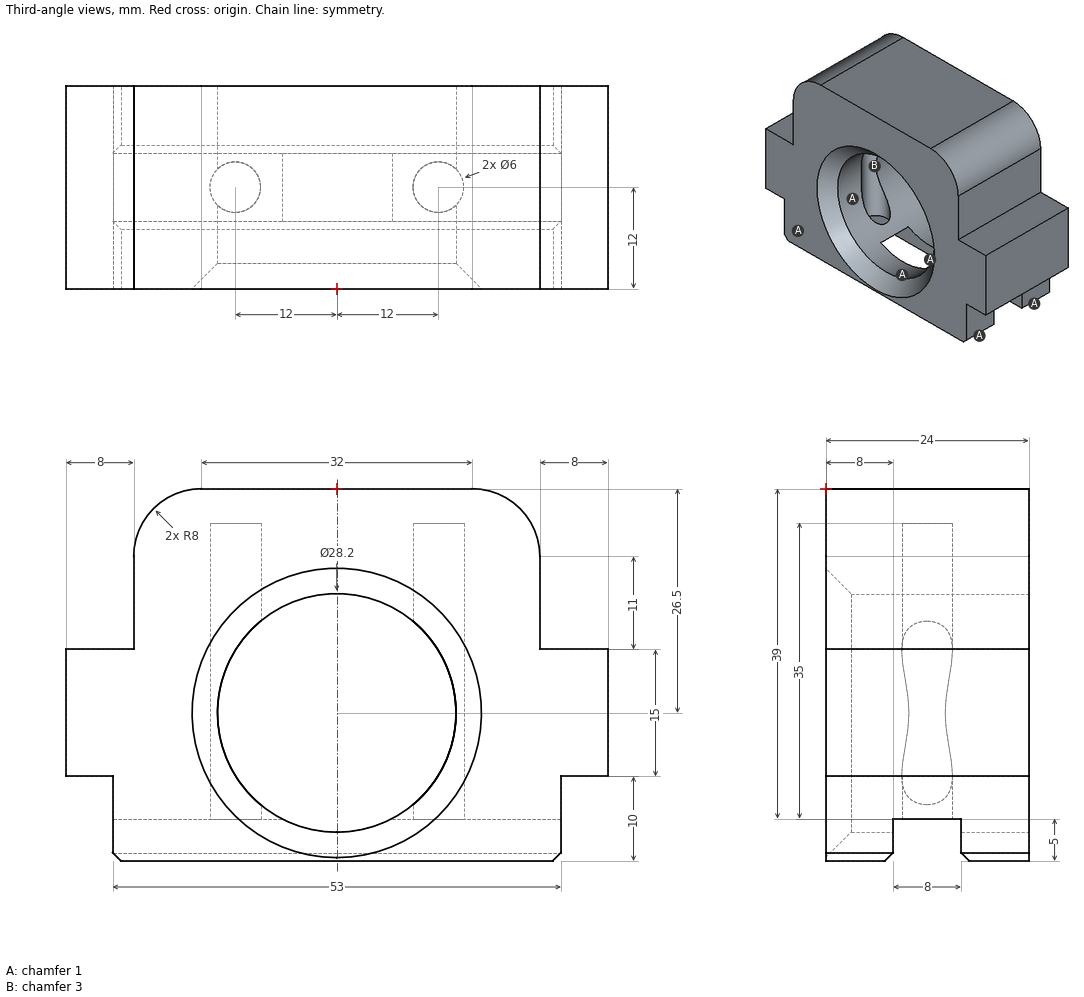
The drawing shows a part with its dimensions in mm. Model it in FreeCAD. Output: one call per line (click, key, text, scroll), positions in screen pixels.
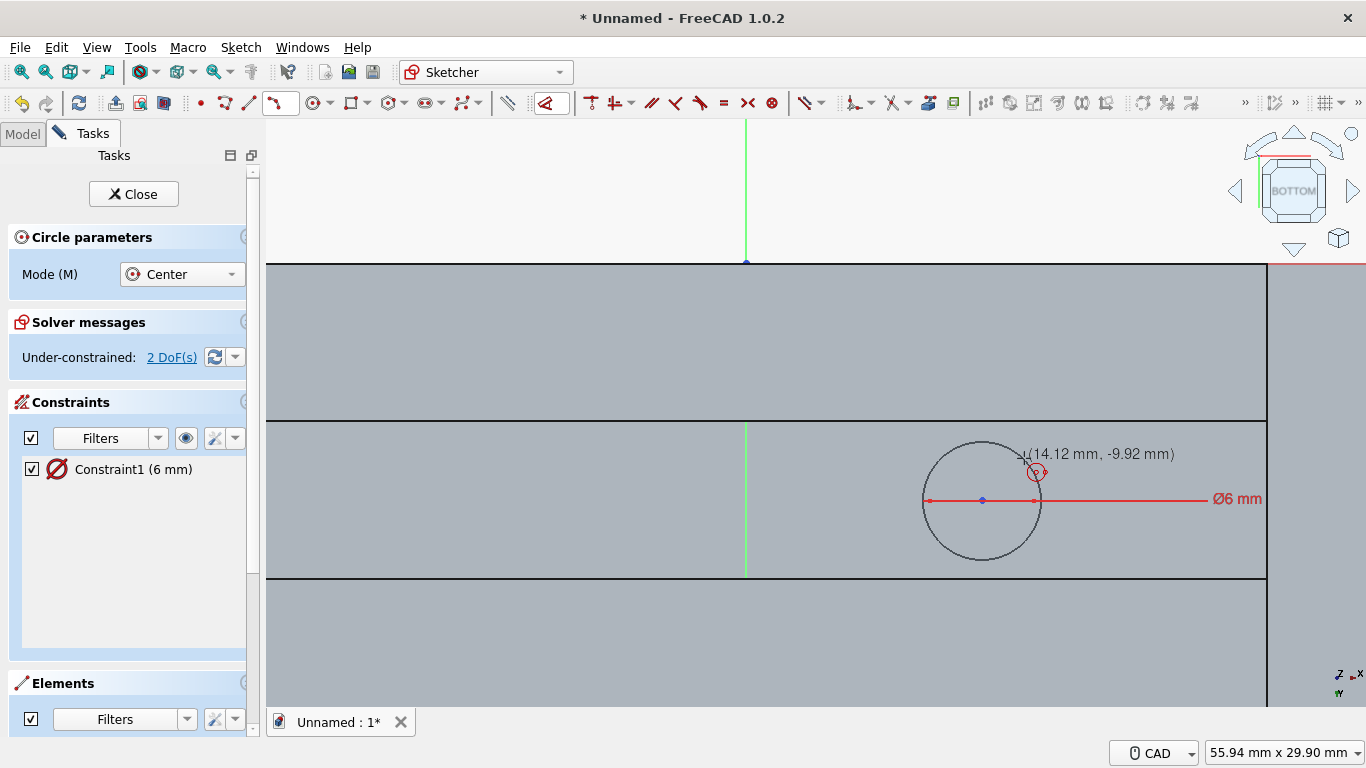
click(510, 500)
move(552, 458)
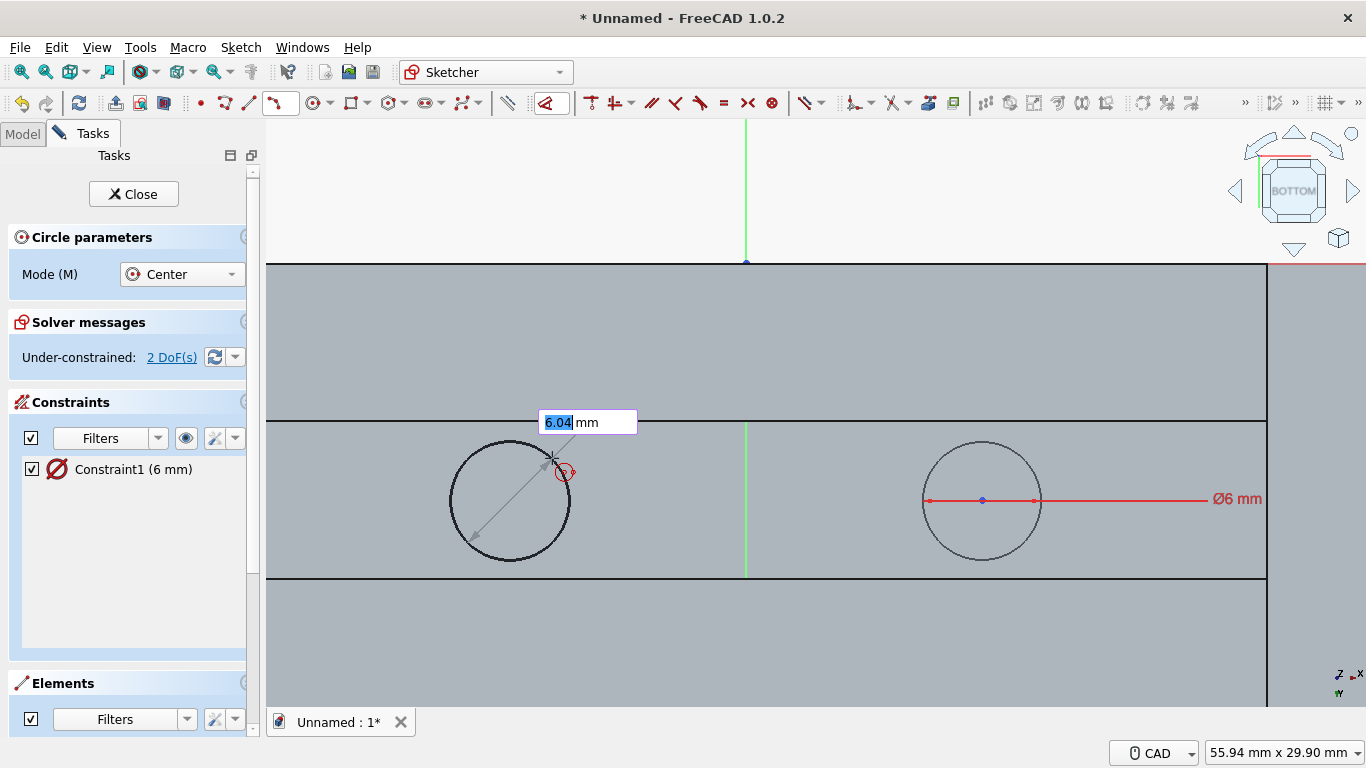
text(6)
key(Return)
key(Escape)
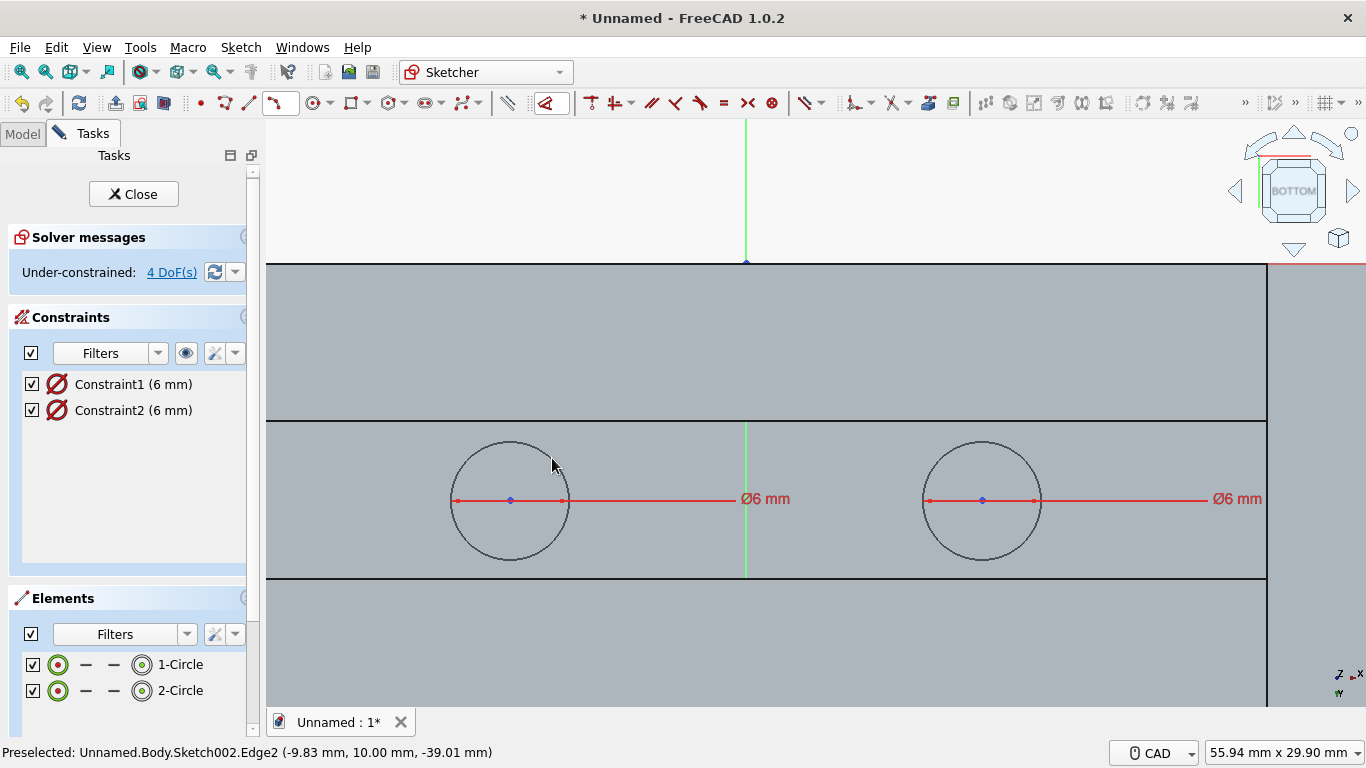
click(982, 501)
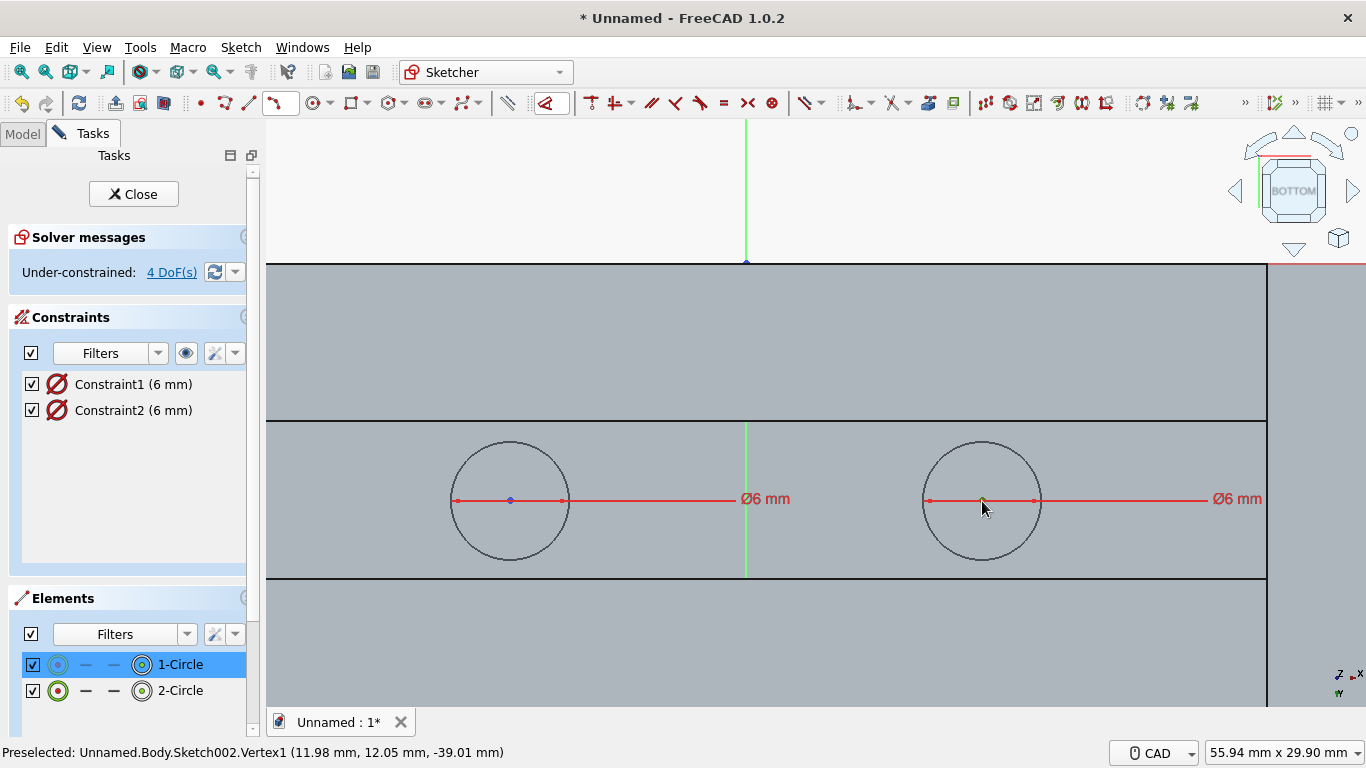
click(510, 501)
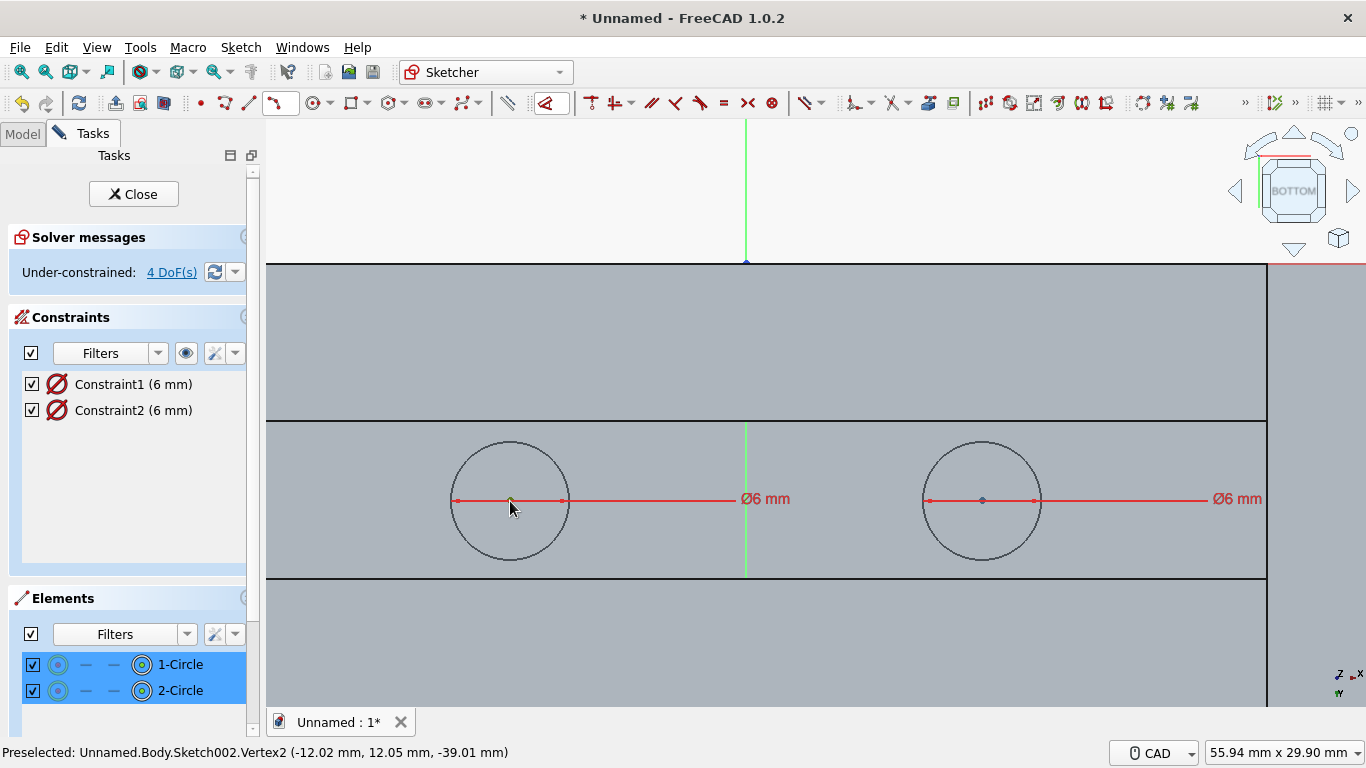
click(634, 104)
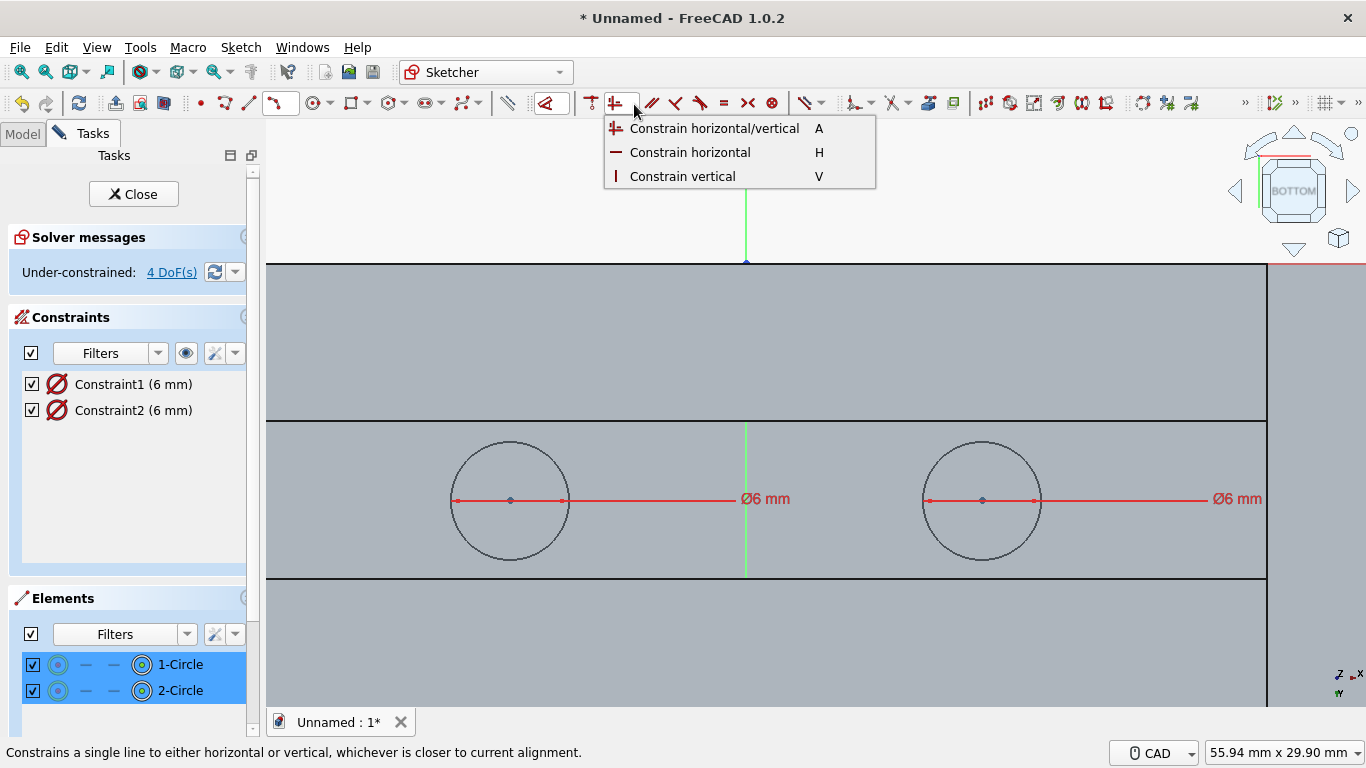
click(740, 152)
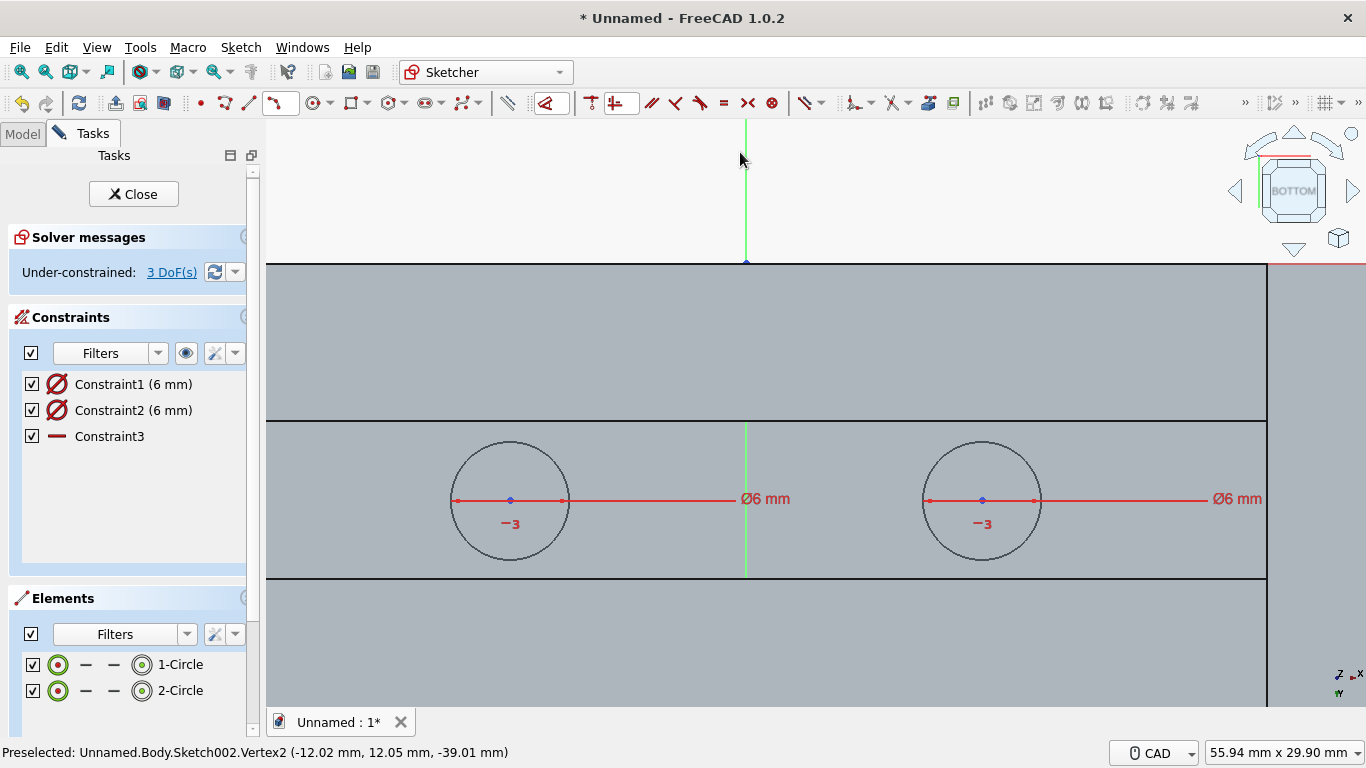
click(982, 501)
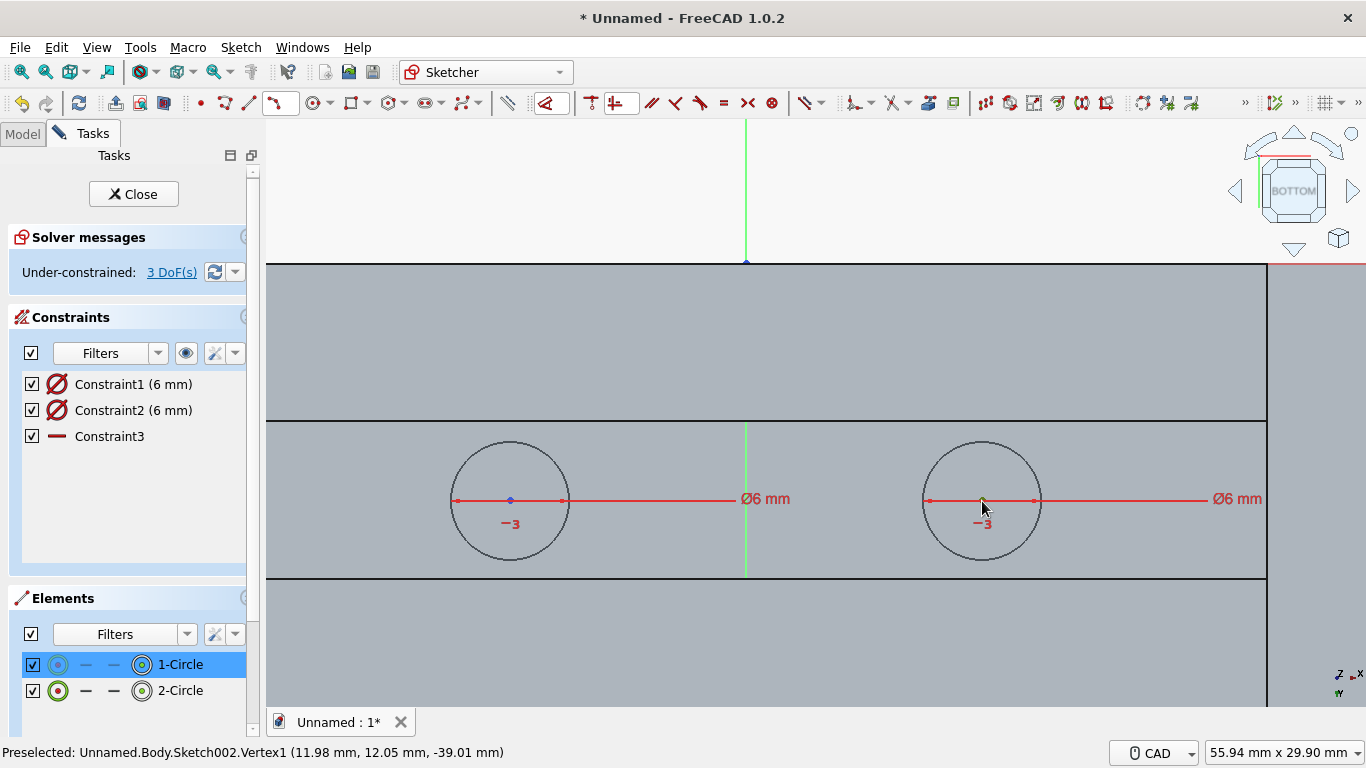
key(l)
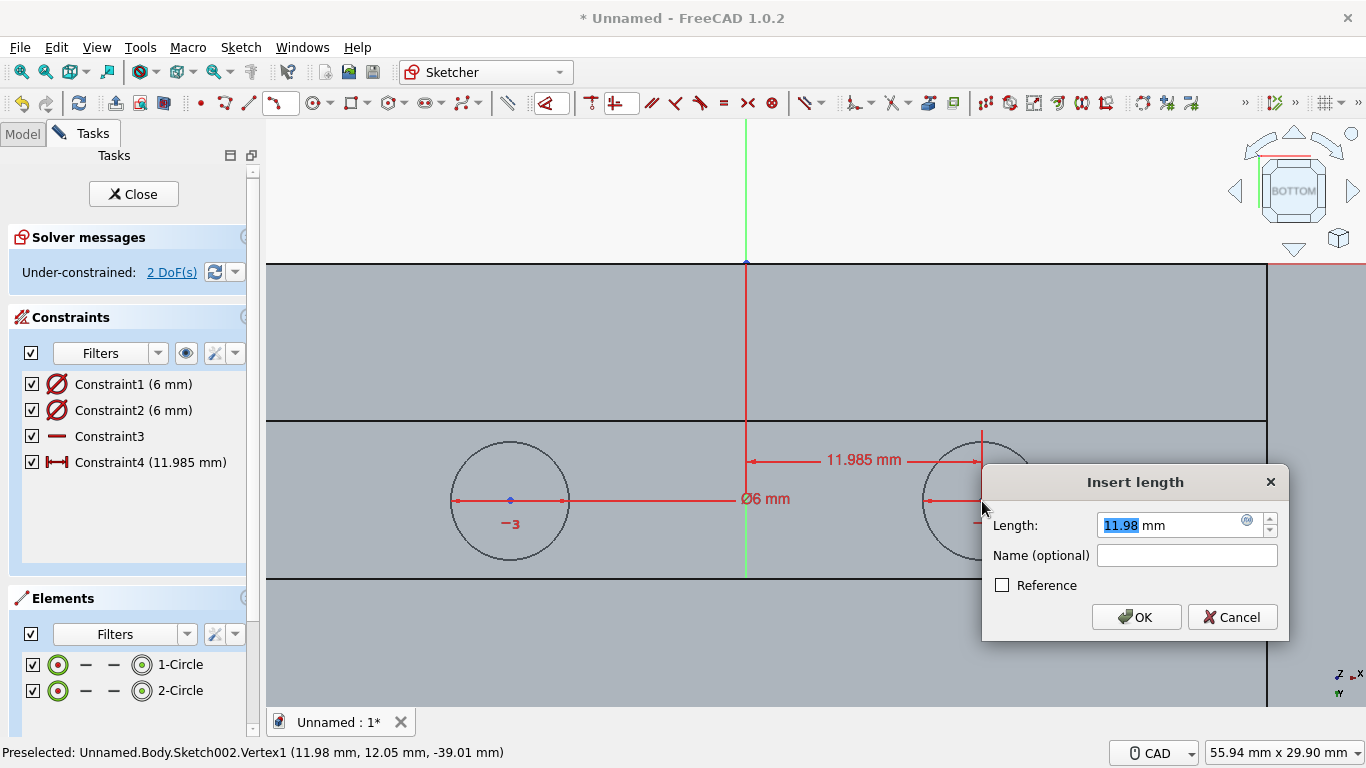
text(12)
key(Return)